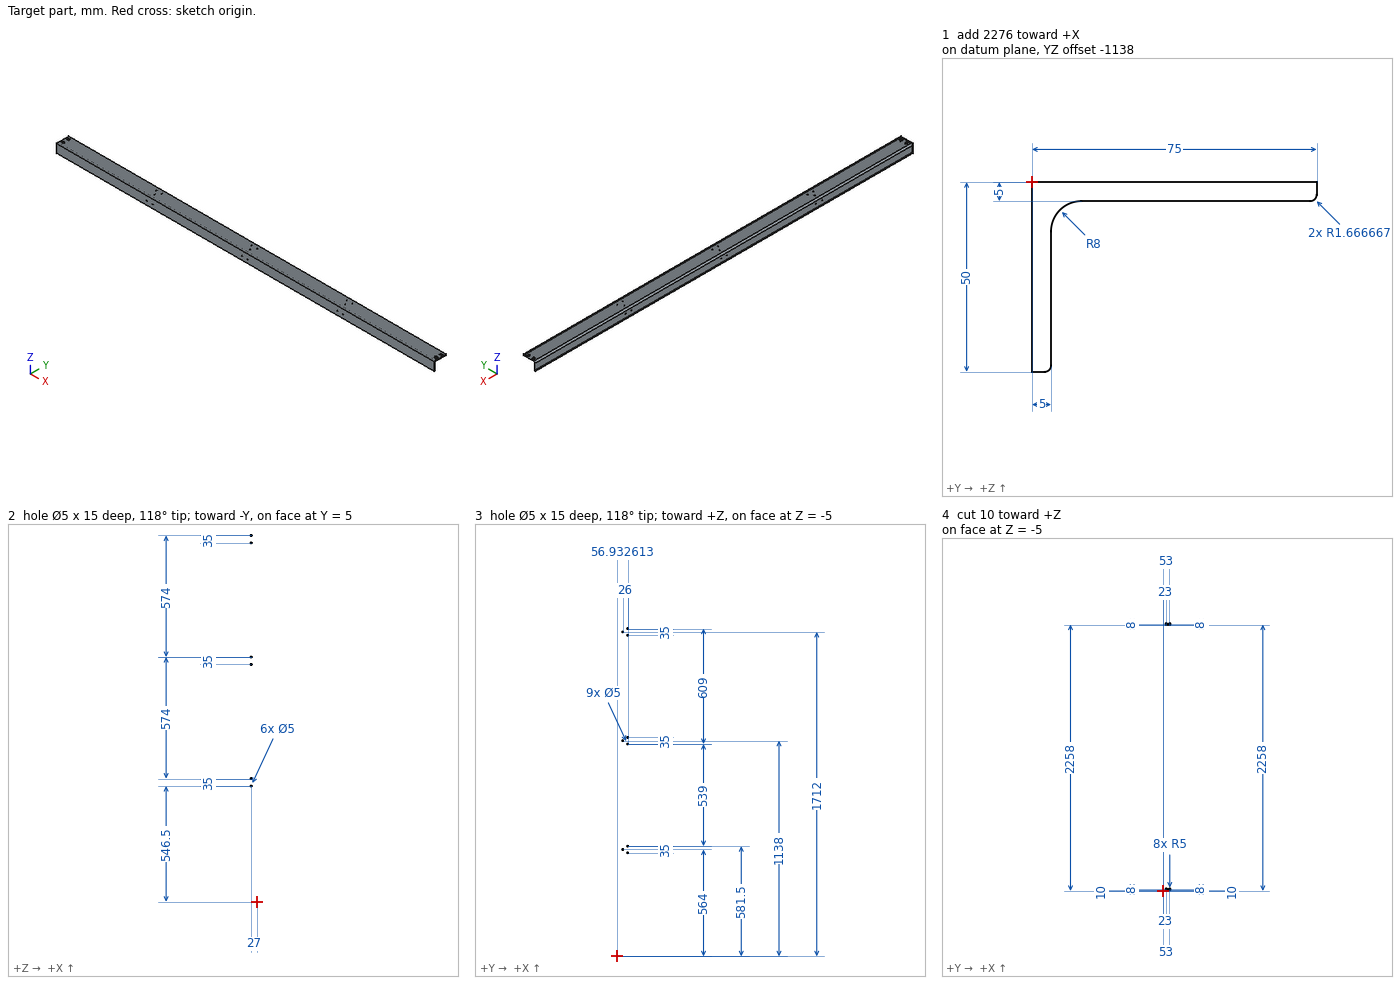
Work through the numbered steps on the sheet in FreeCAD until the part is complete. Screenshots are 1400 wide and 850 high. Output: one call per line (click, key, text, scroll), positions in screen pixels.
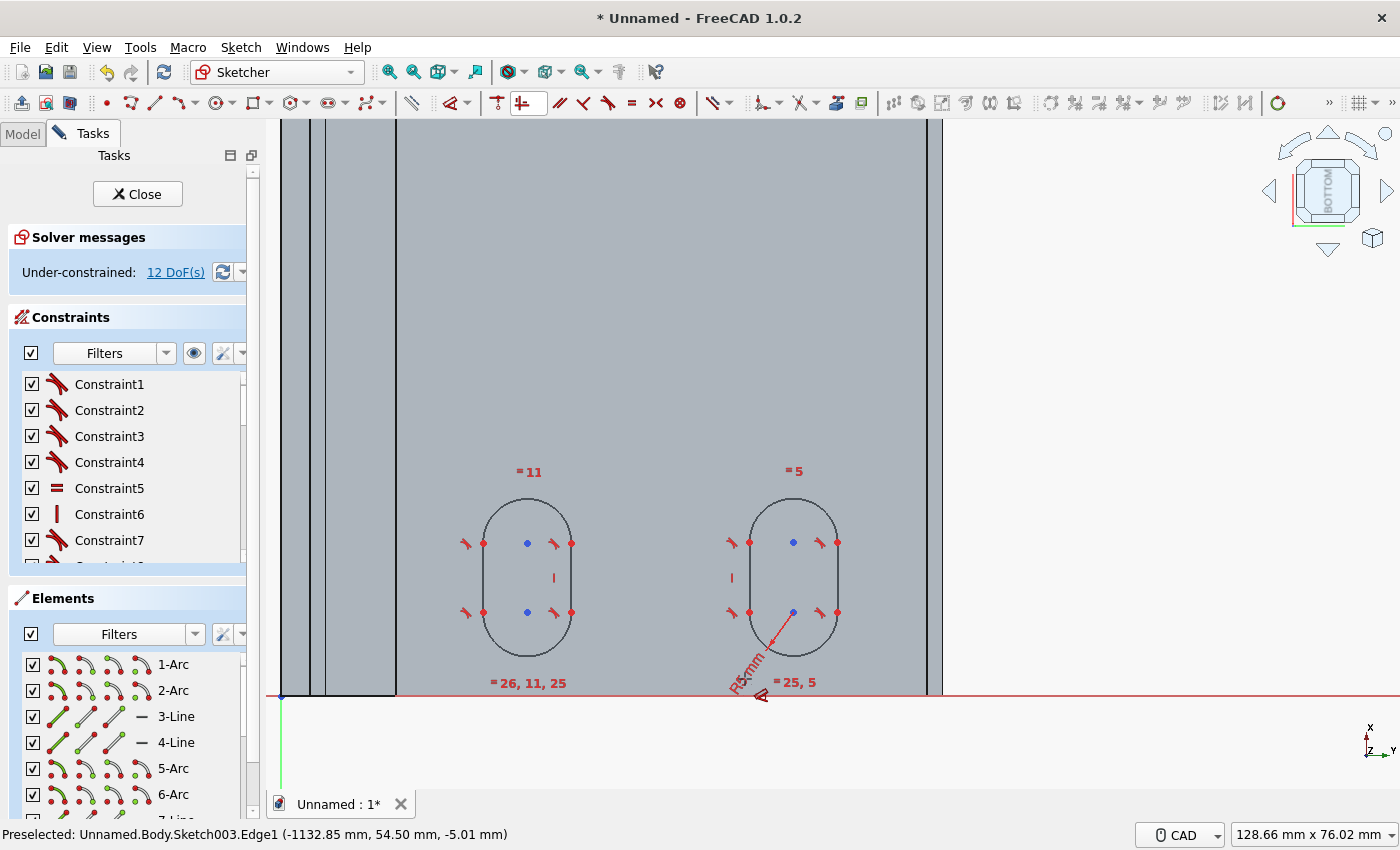
click(750, 591)
click(784, 577)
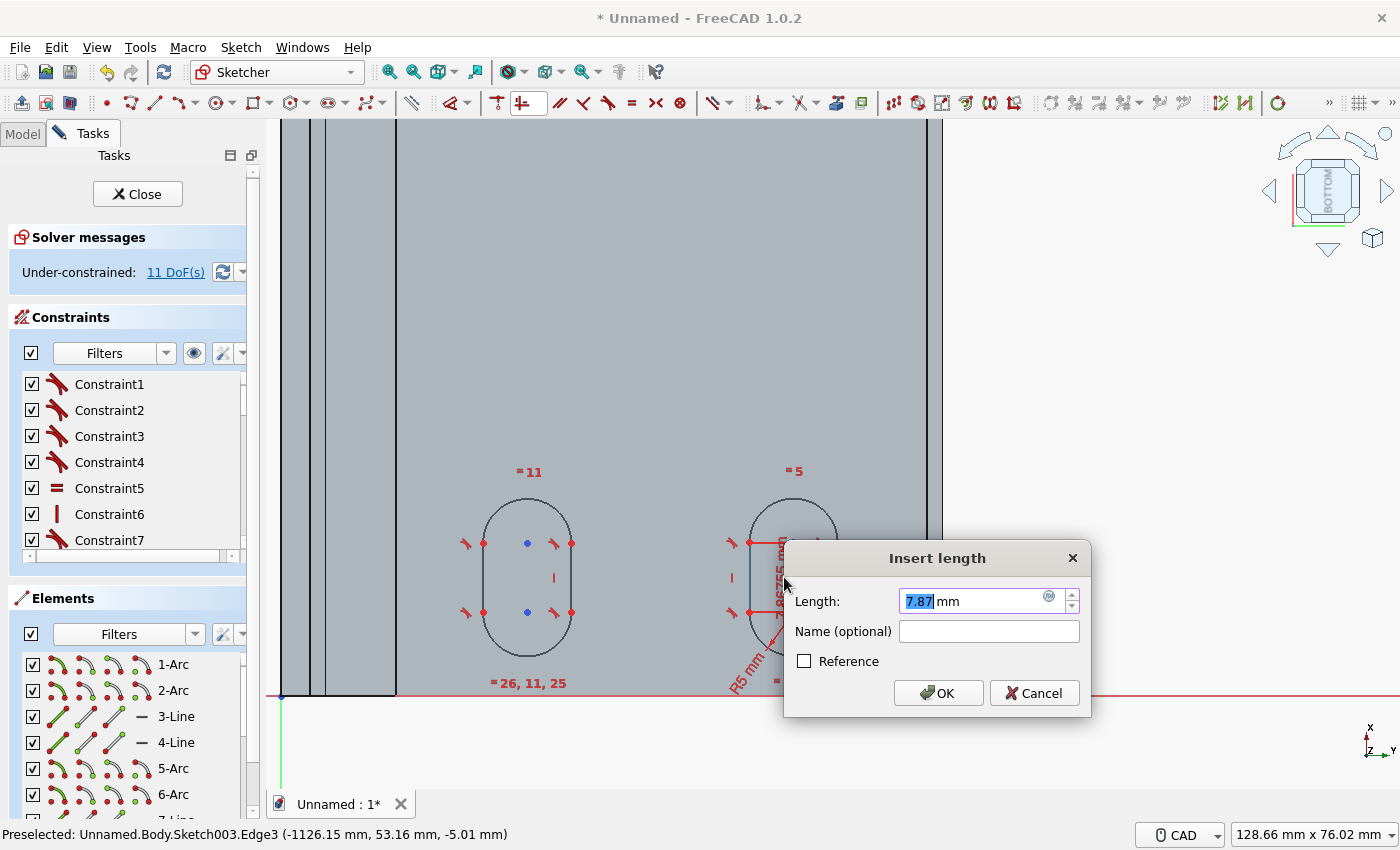
text(8)
key(Return)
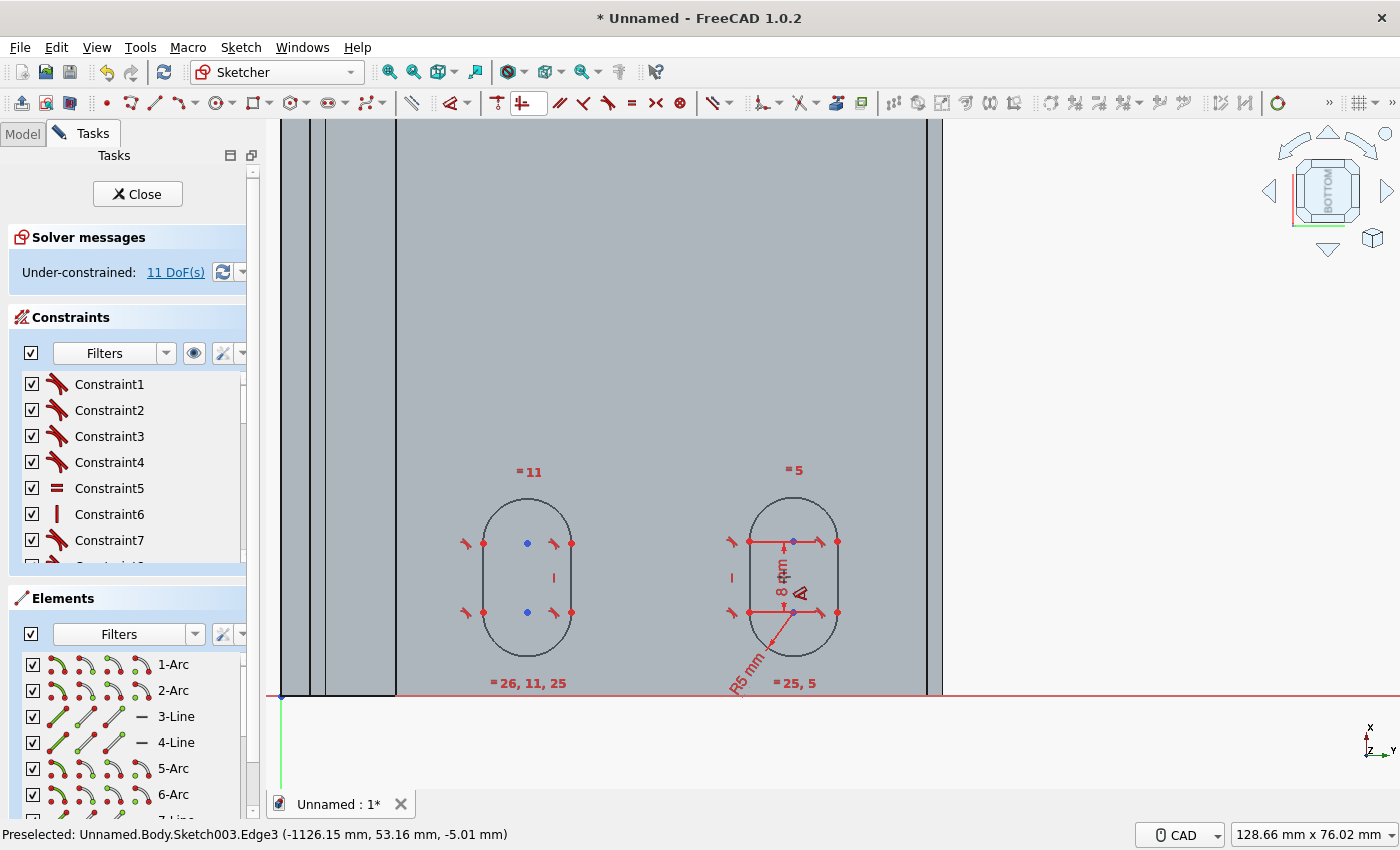
click(483, 592)
click(449, 578)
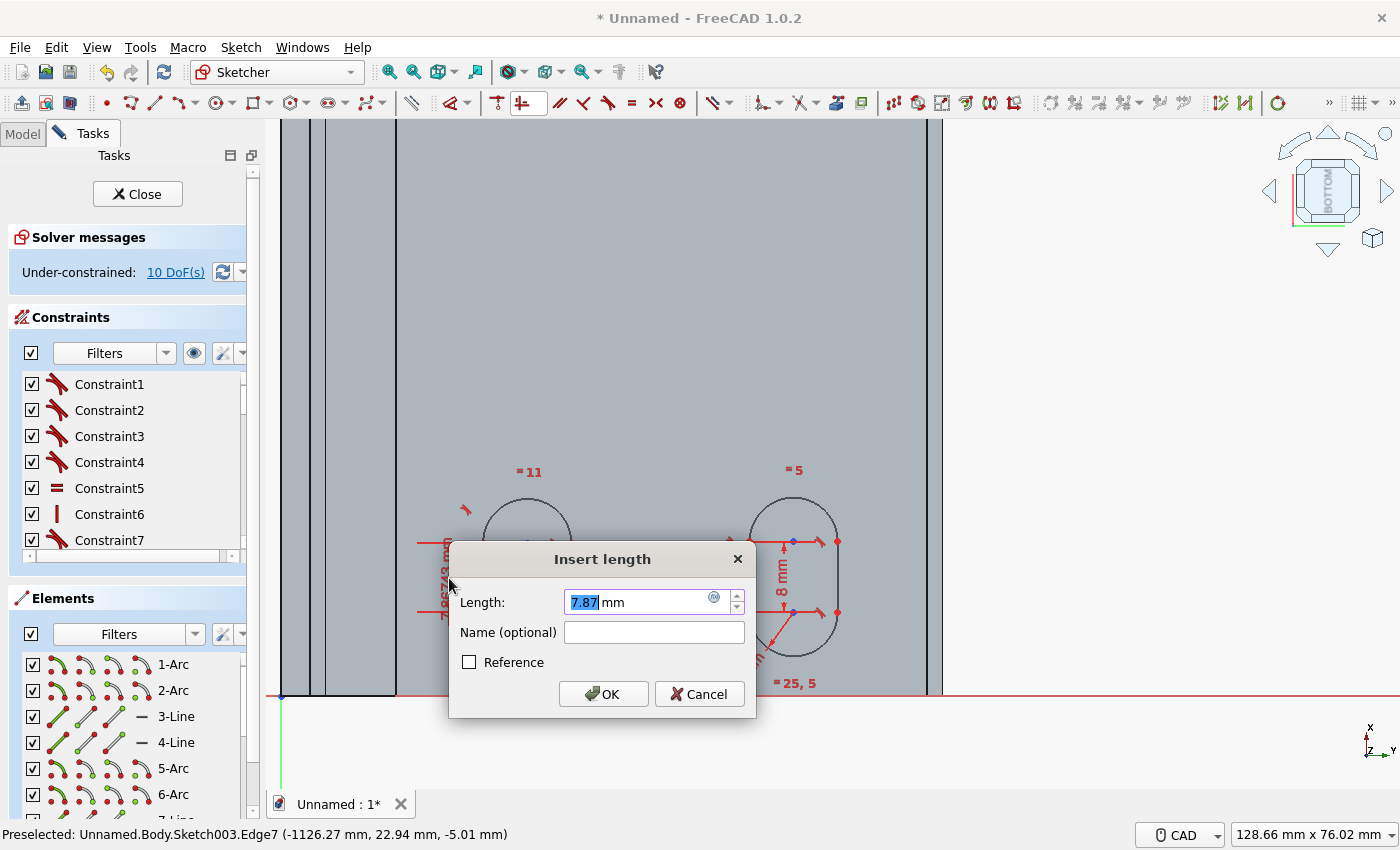
text(8)
key(Return)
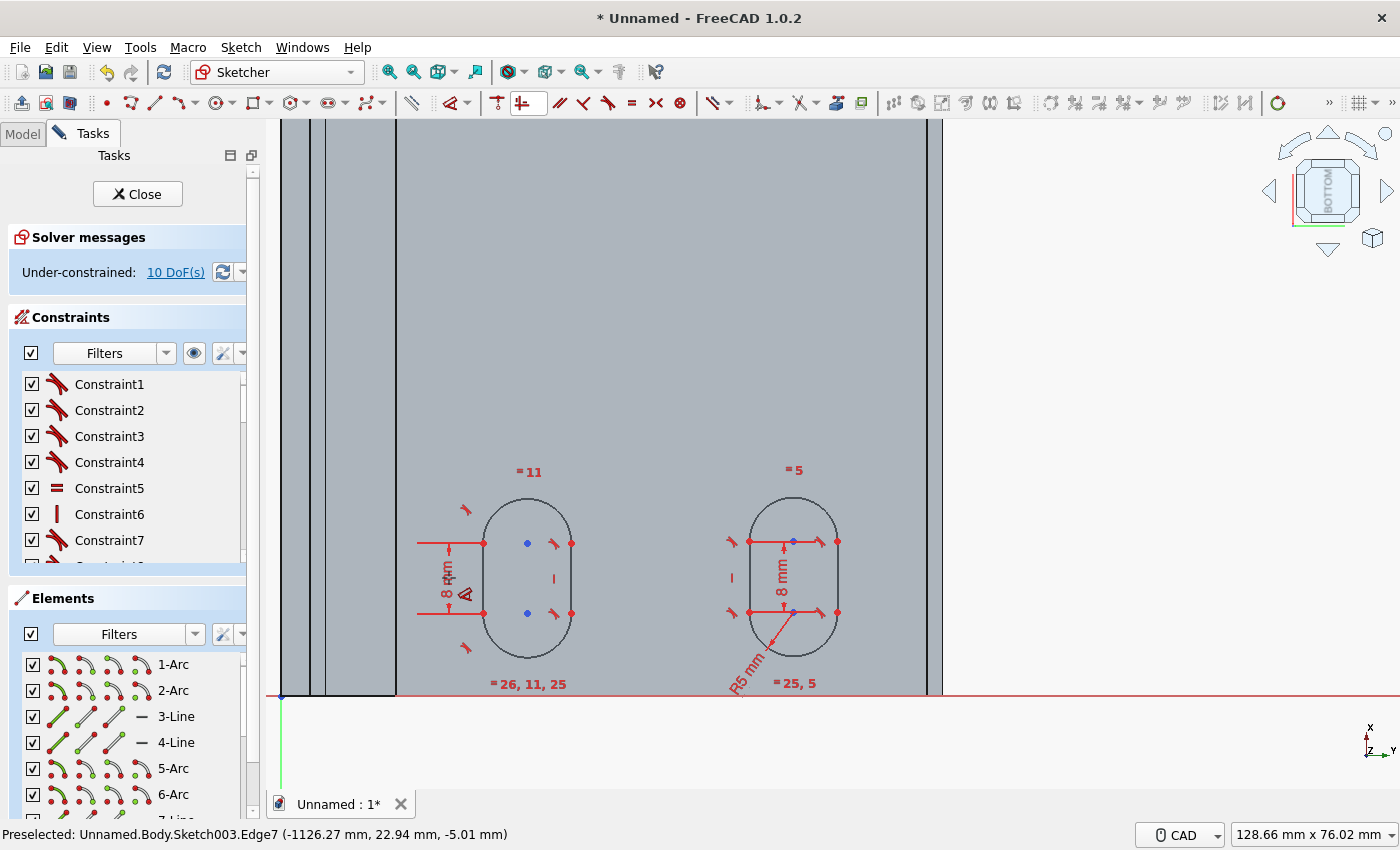
scroll(770, 728, down, 18)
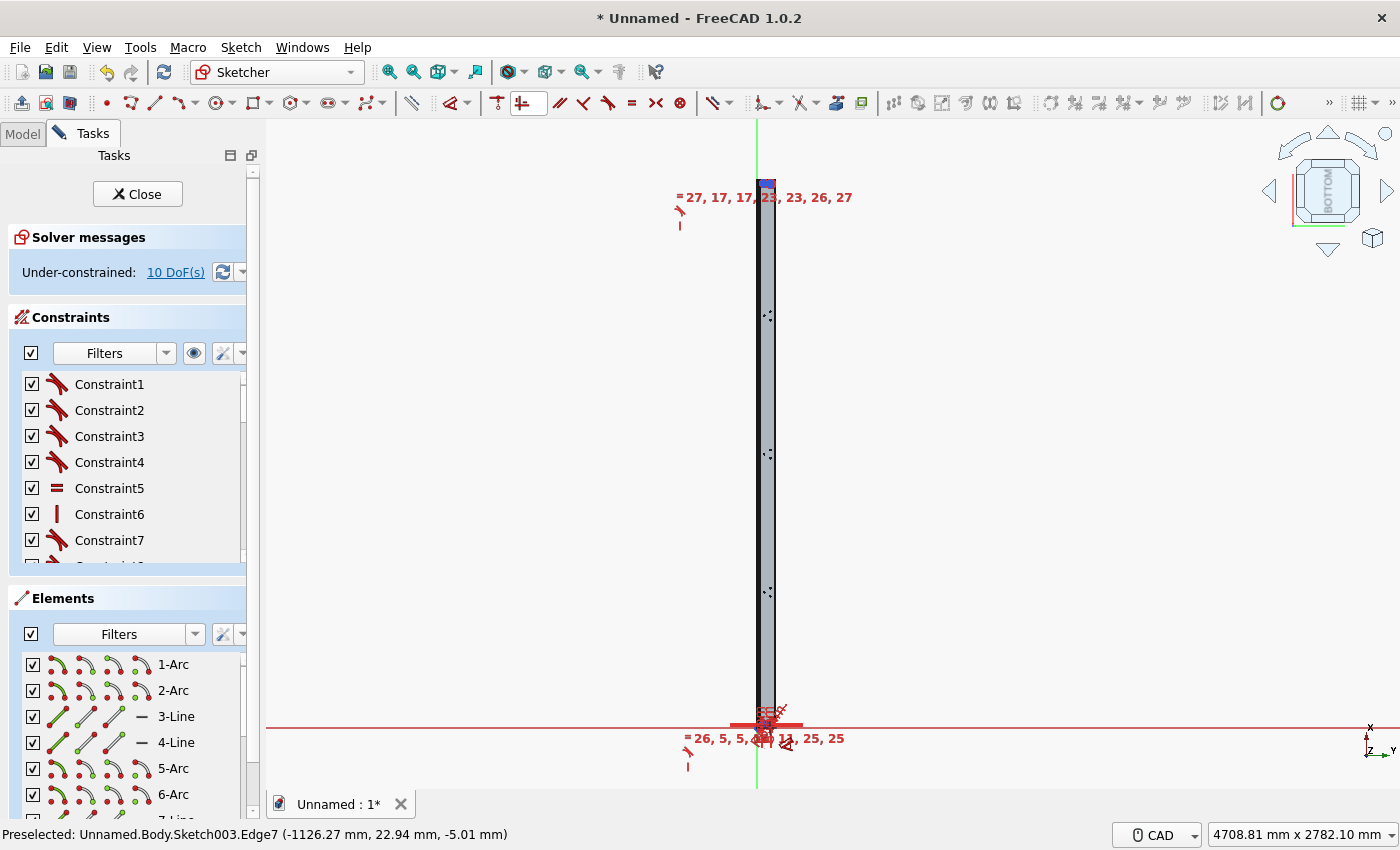
scroll(770, 184, up, 16)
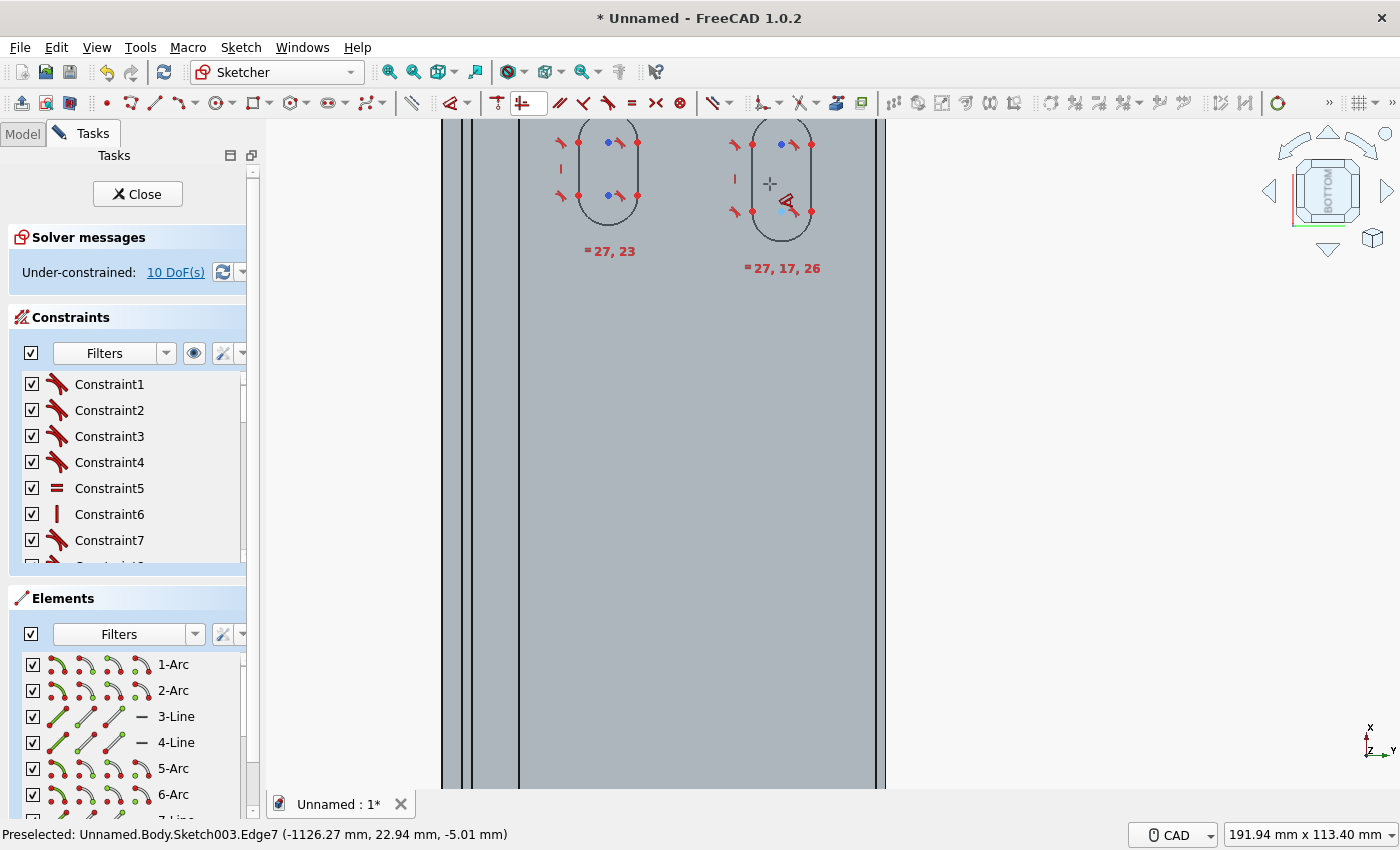
click(752, 192)
click(786, 179)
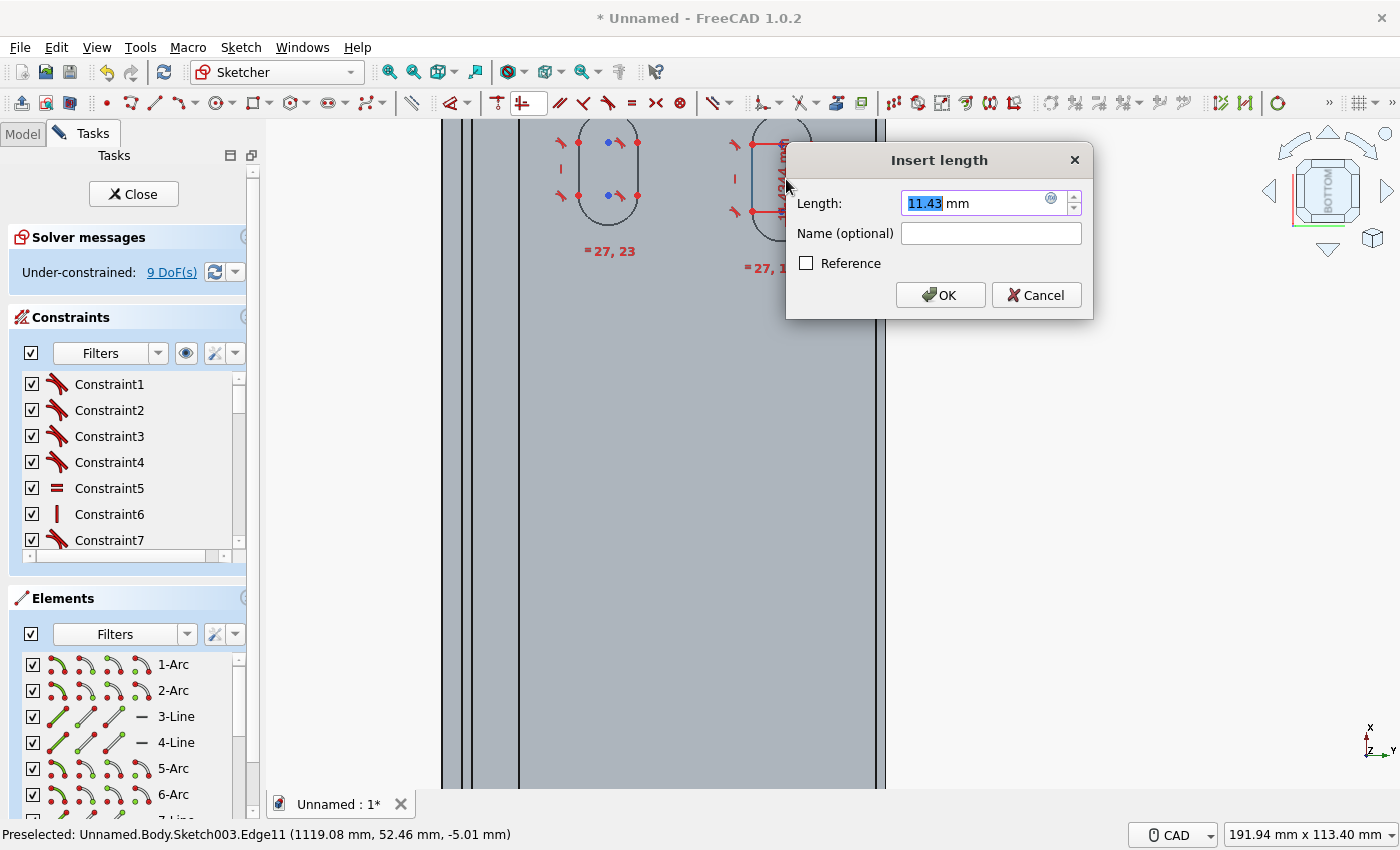
text(8)
key(Return)